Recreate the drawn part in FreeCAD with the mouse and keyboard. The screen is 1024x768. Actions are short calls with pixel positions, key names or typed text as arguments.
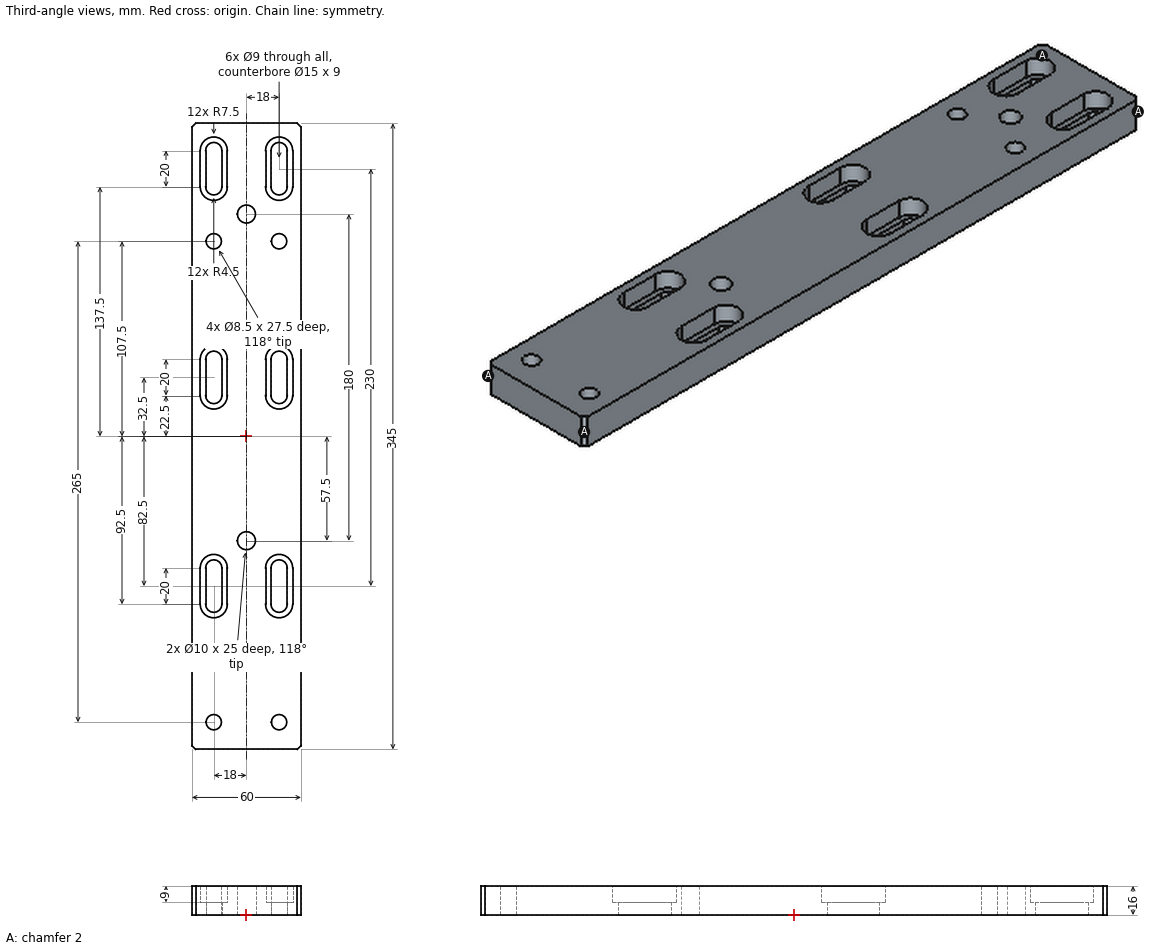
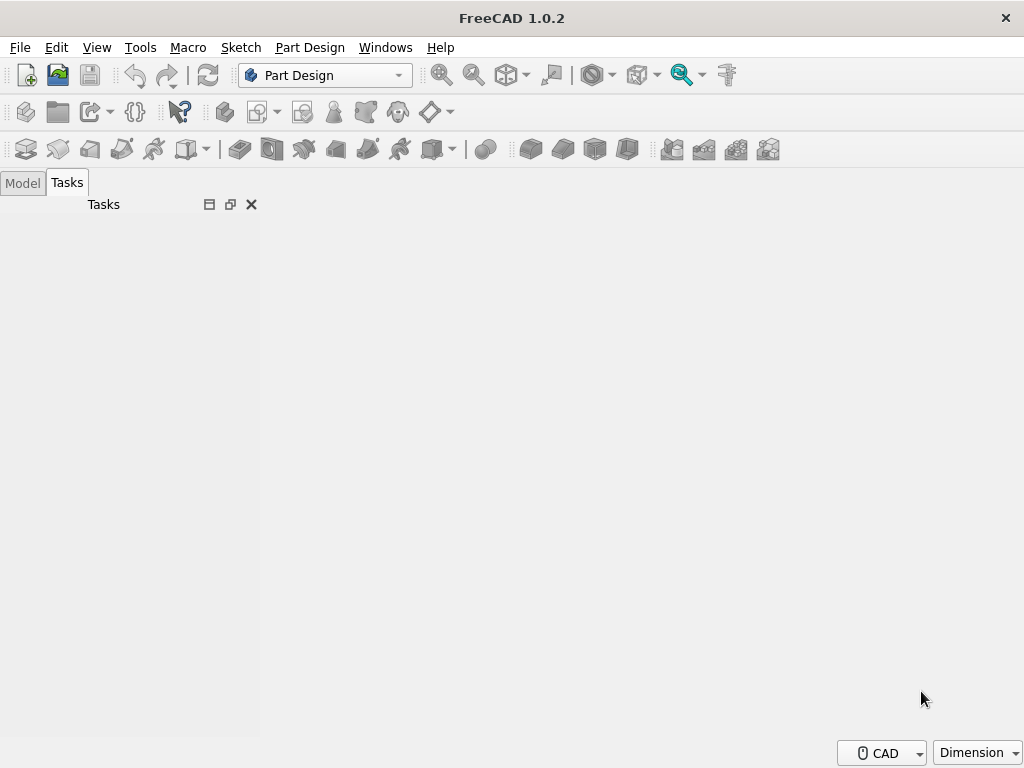
key(ctrl+n)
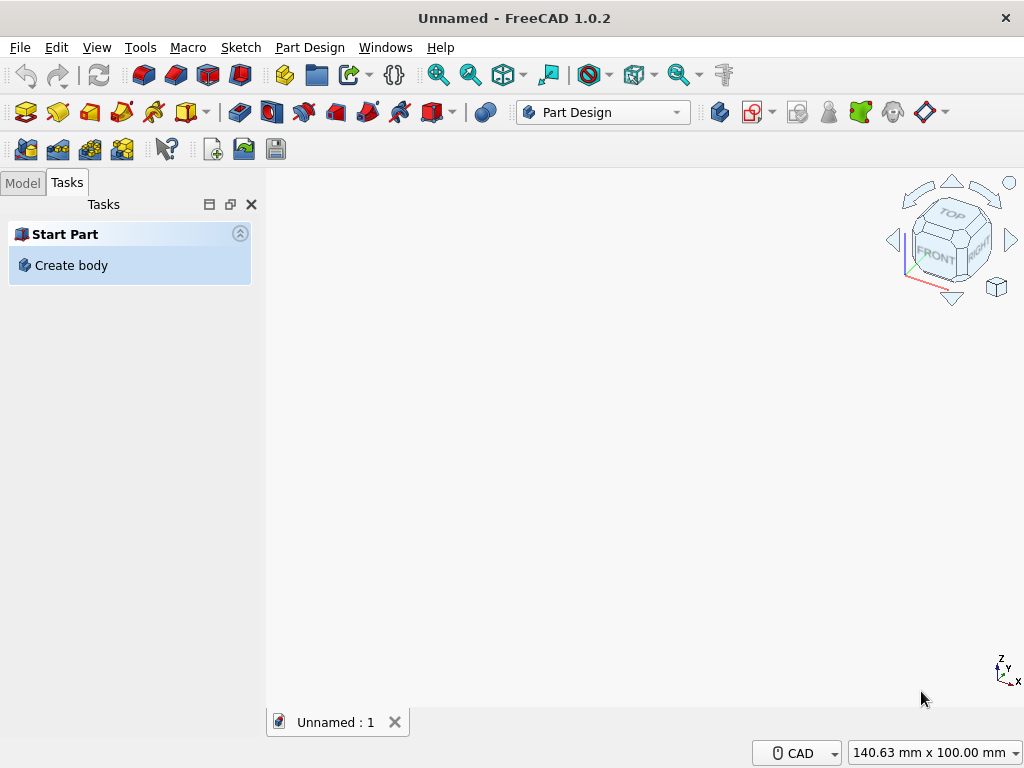
click(752, 112)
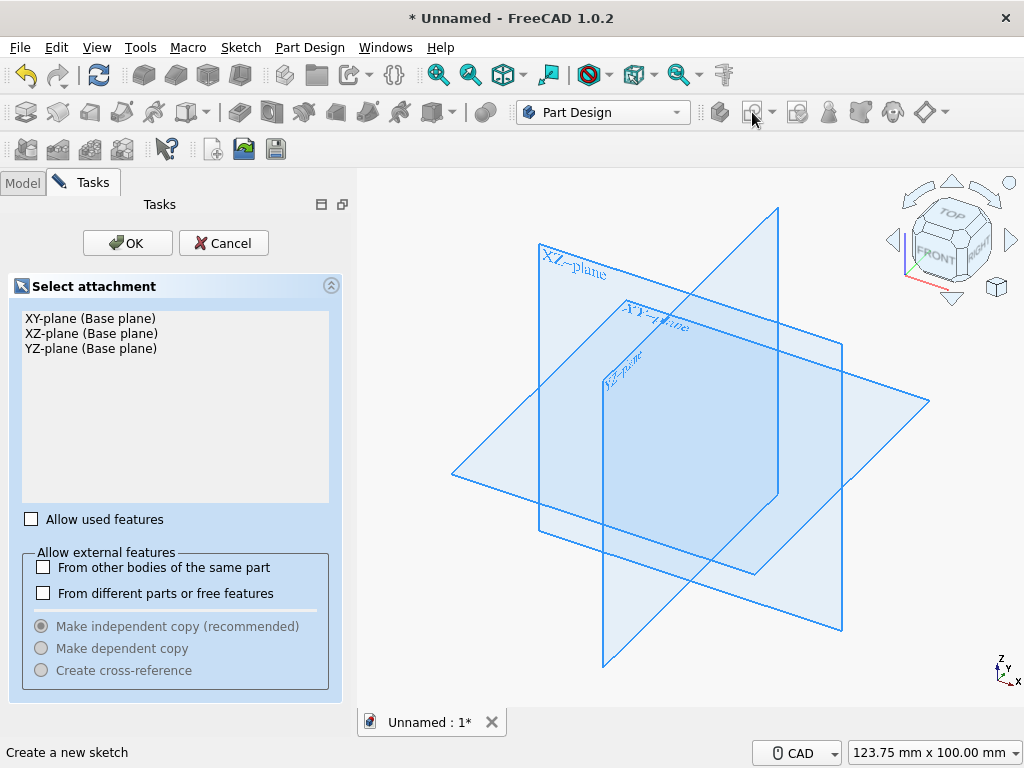
click(82, 318)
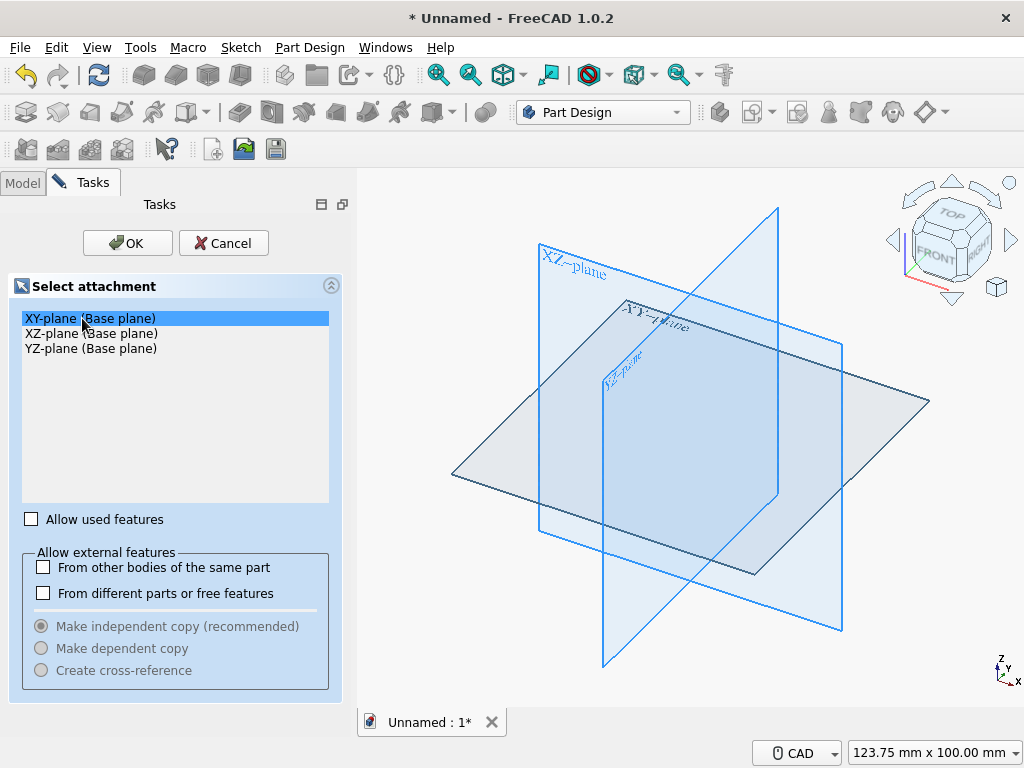
click(128, 243)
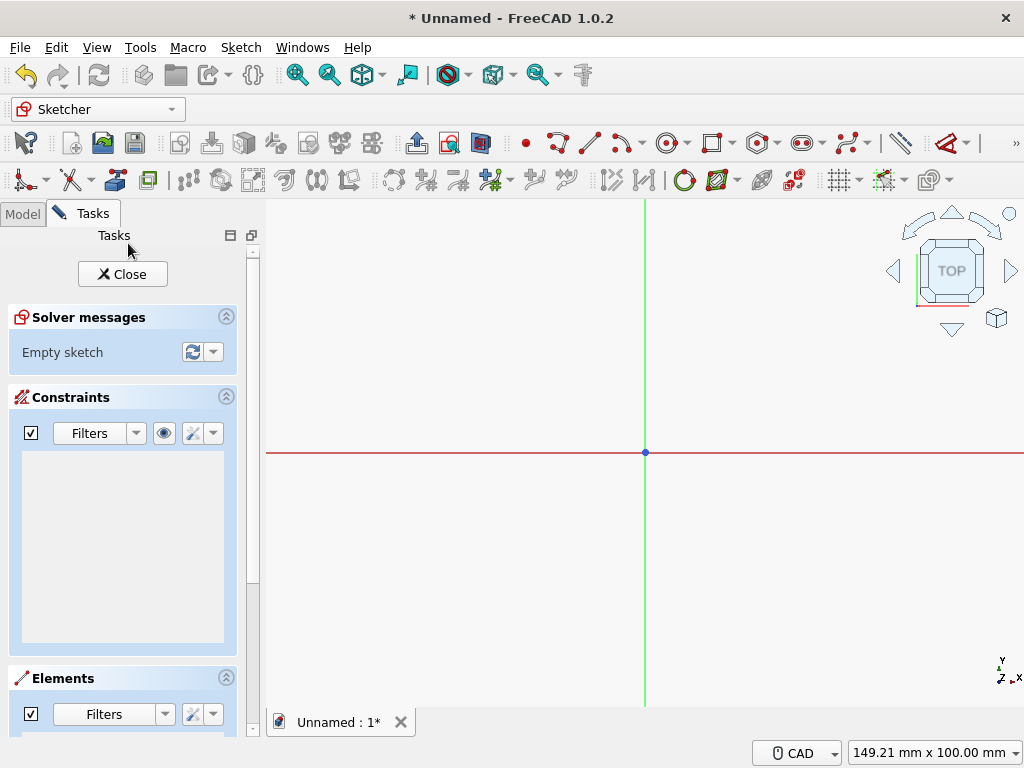
scroll(563, 453, down, 9)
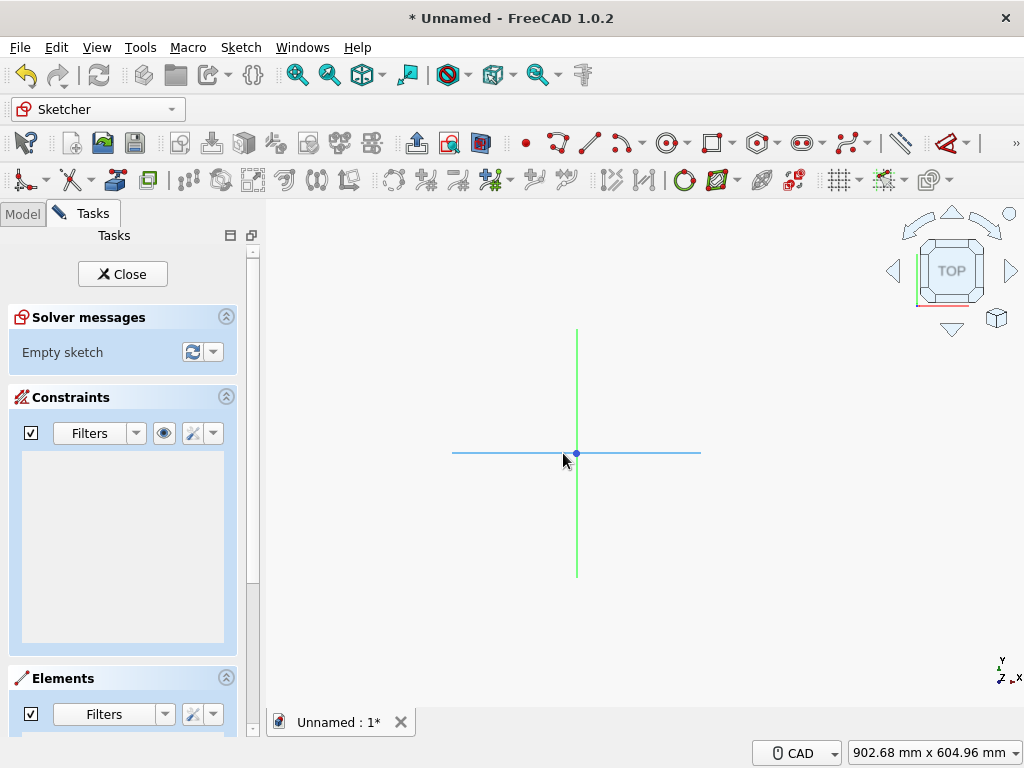
click(734, 144)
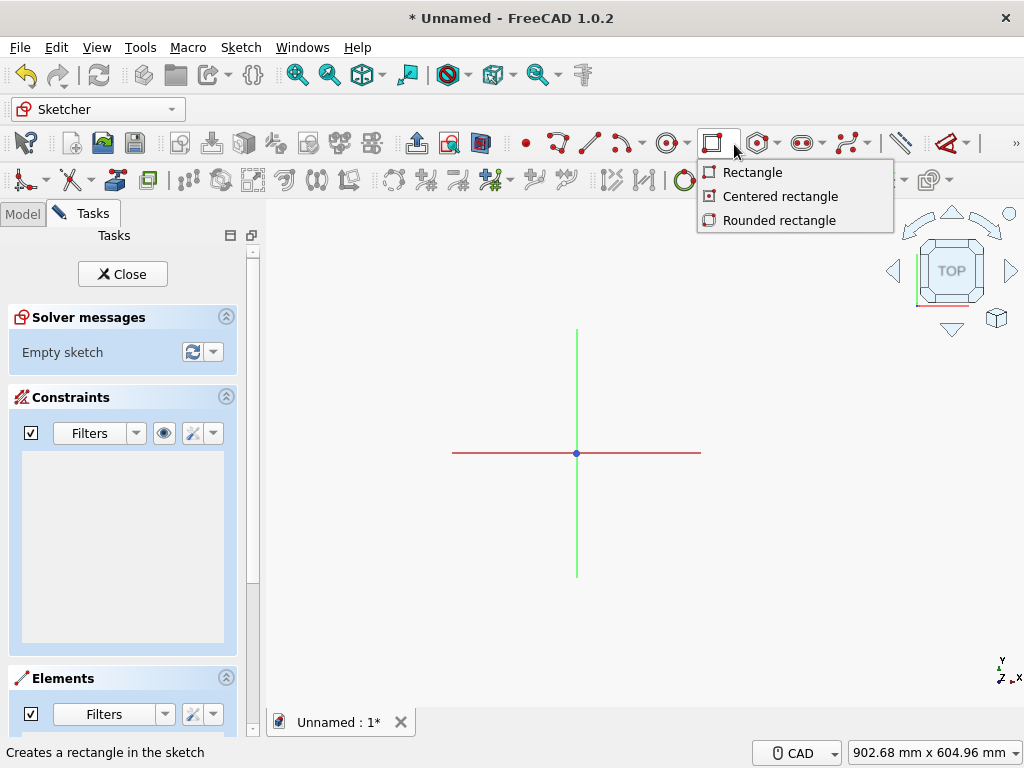
click(796, 196)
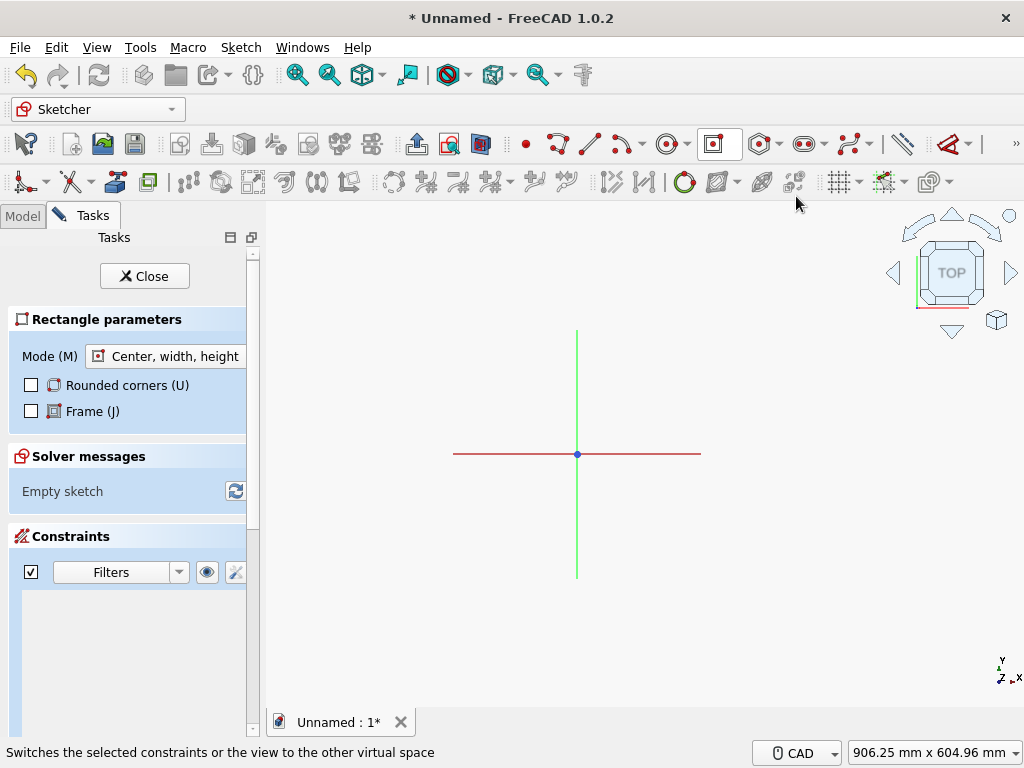
click(577, 454)
click(602, 310)
key(Escape)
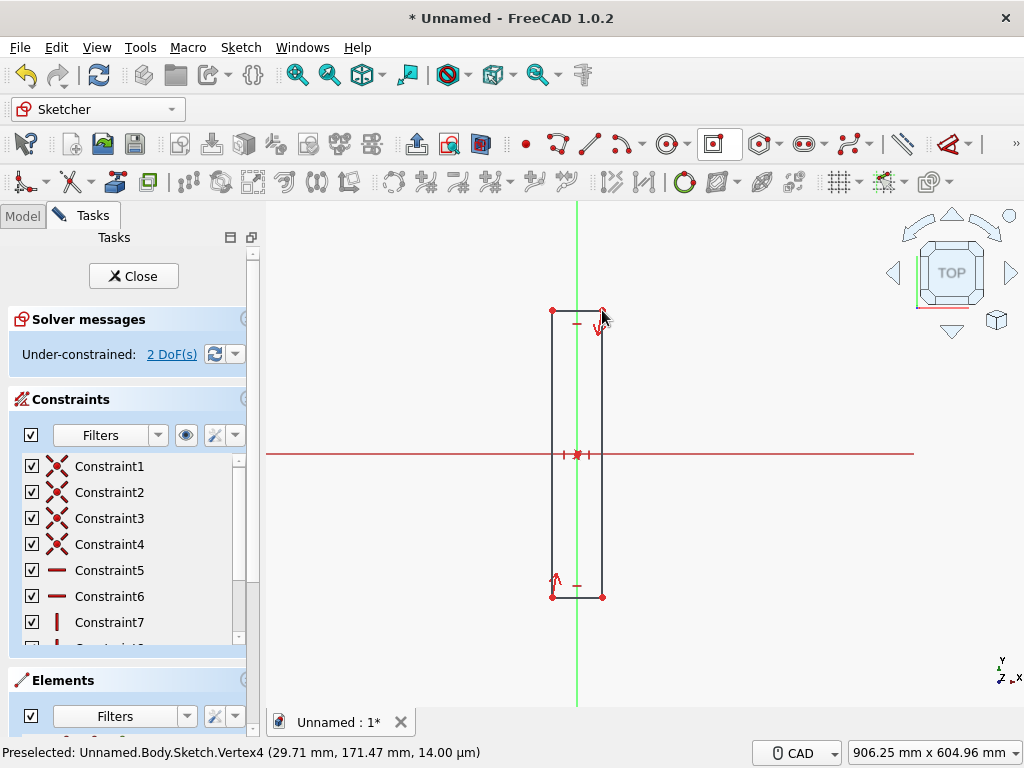
key(d)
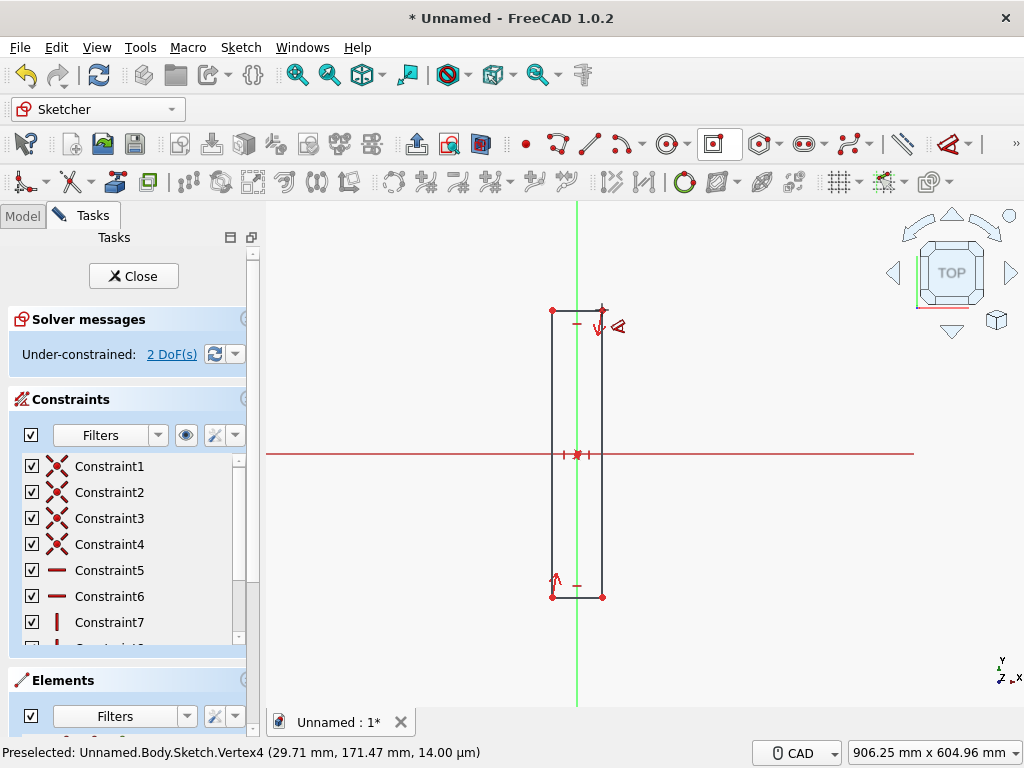
scroll(567, 598, up, 2)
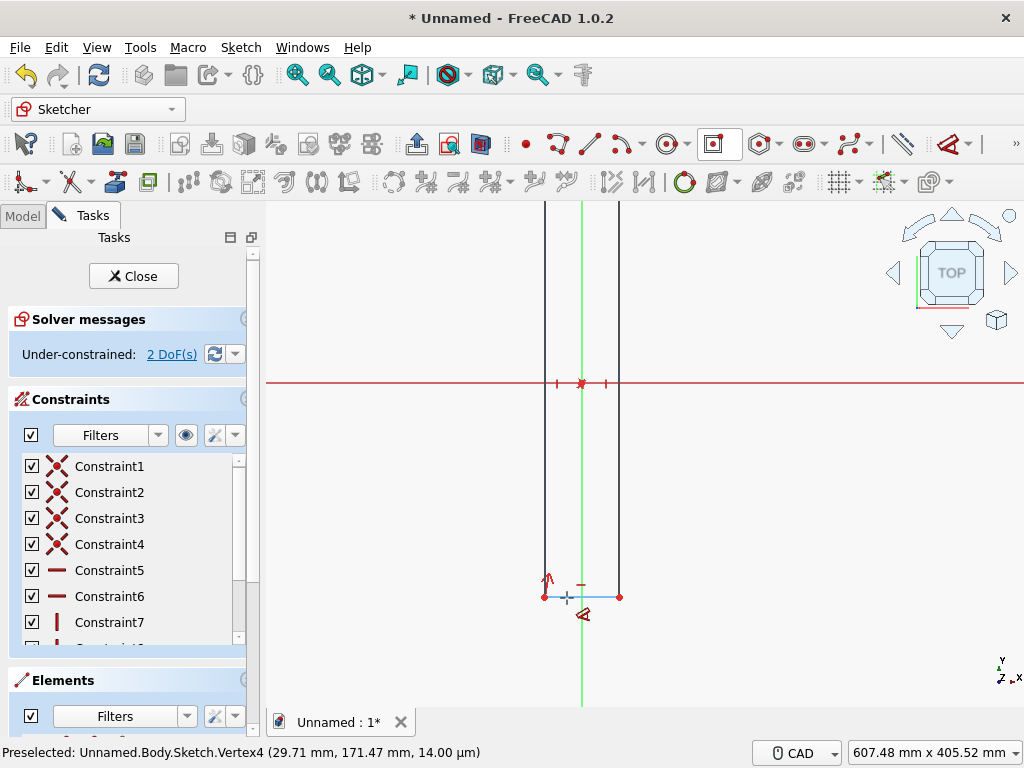
click(567, 597)
click(565, 631)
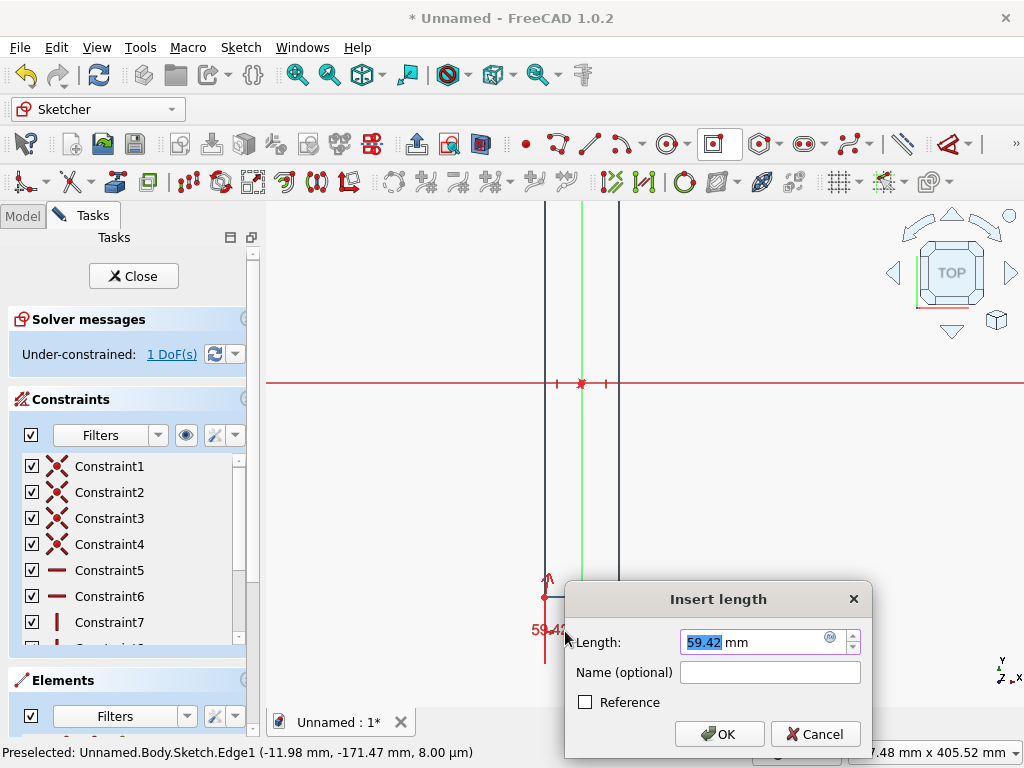
text(60)
key(Return)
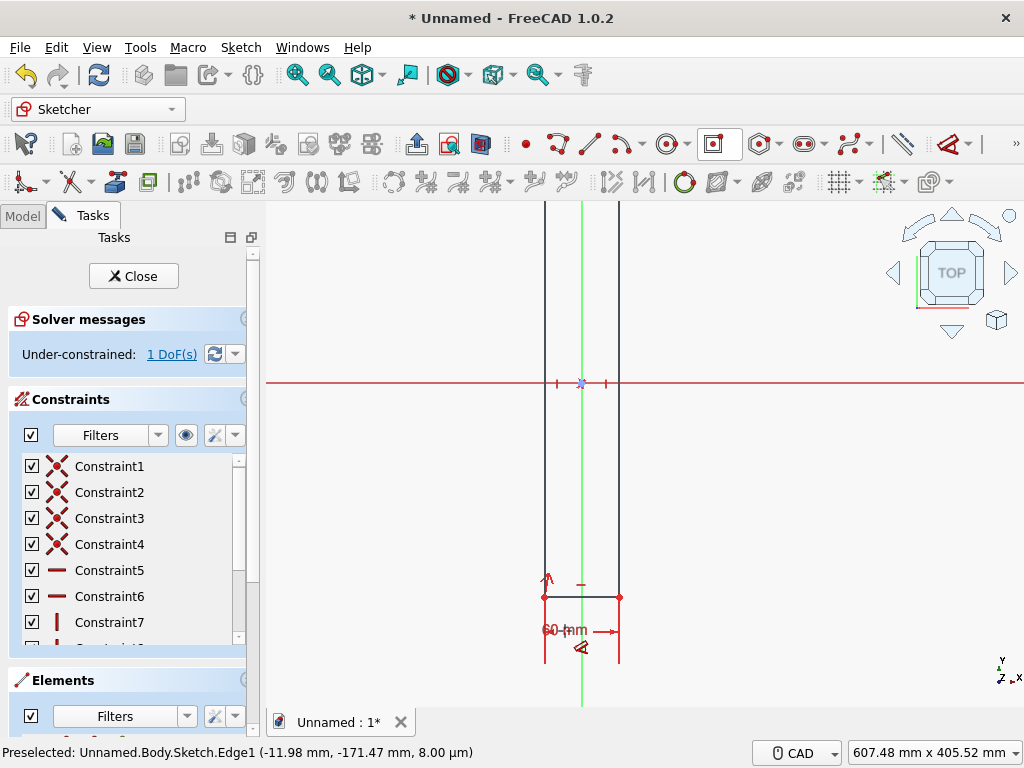
click(619, 469)
click(653, 413)